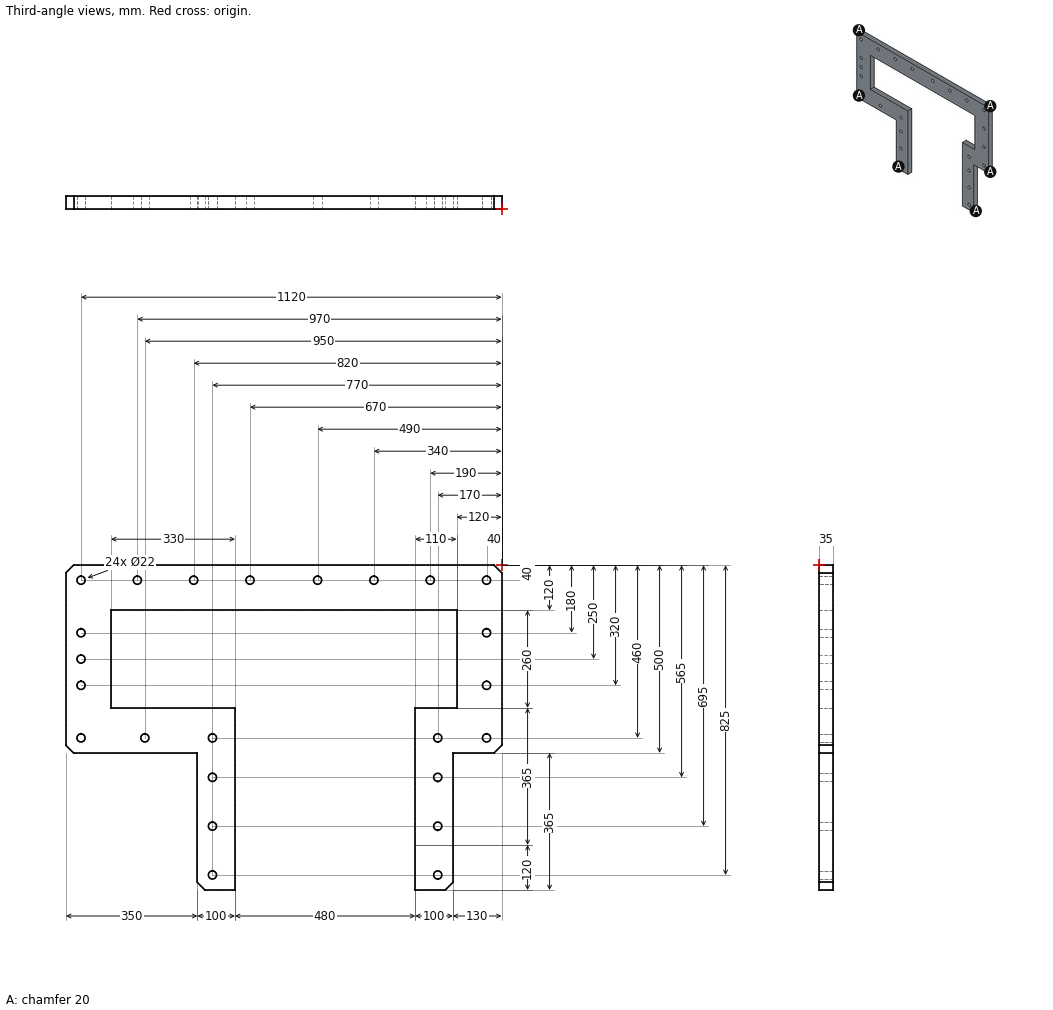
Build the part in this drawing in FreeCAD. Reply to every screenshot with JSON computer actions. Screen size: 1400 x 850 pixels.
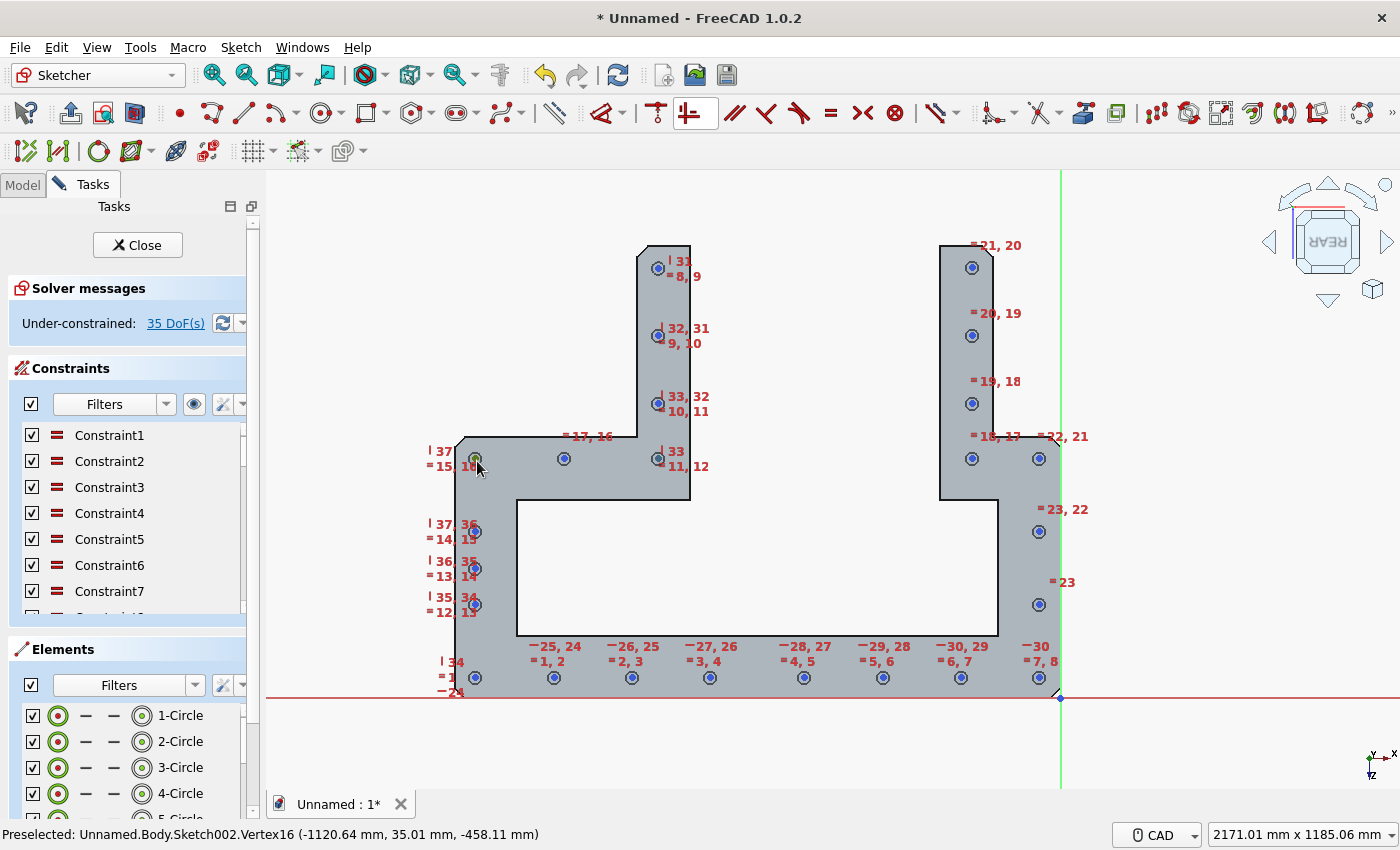
{"action": "key", "text": "h"}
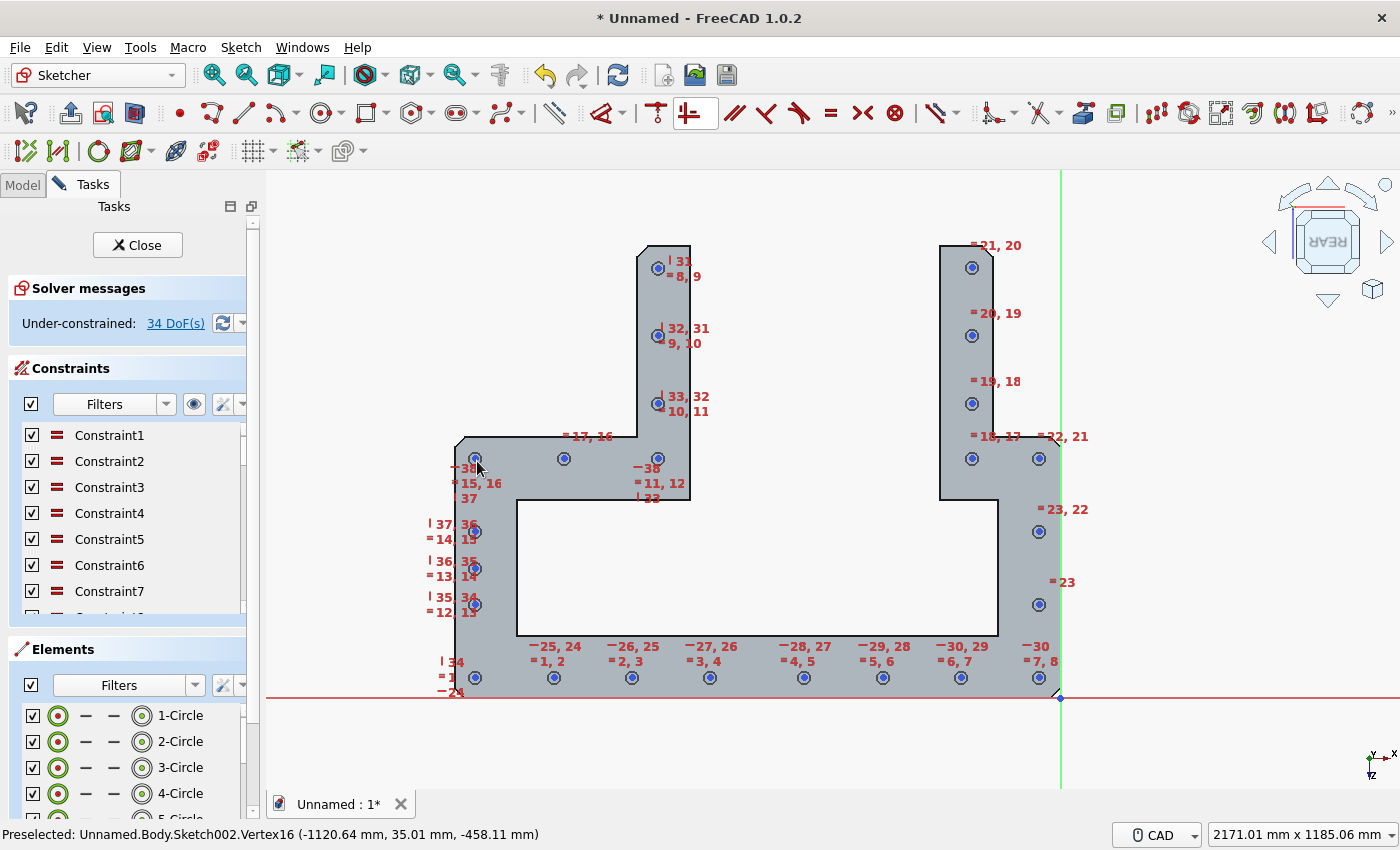
{"action": "left_click", "coordinate": [475, 459]}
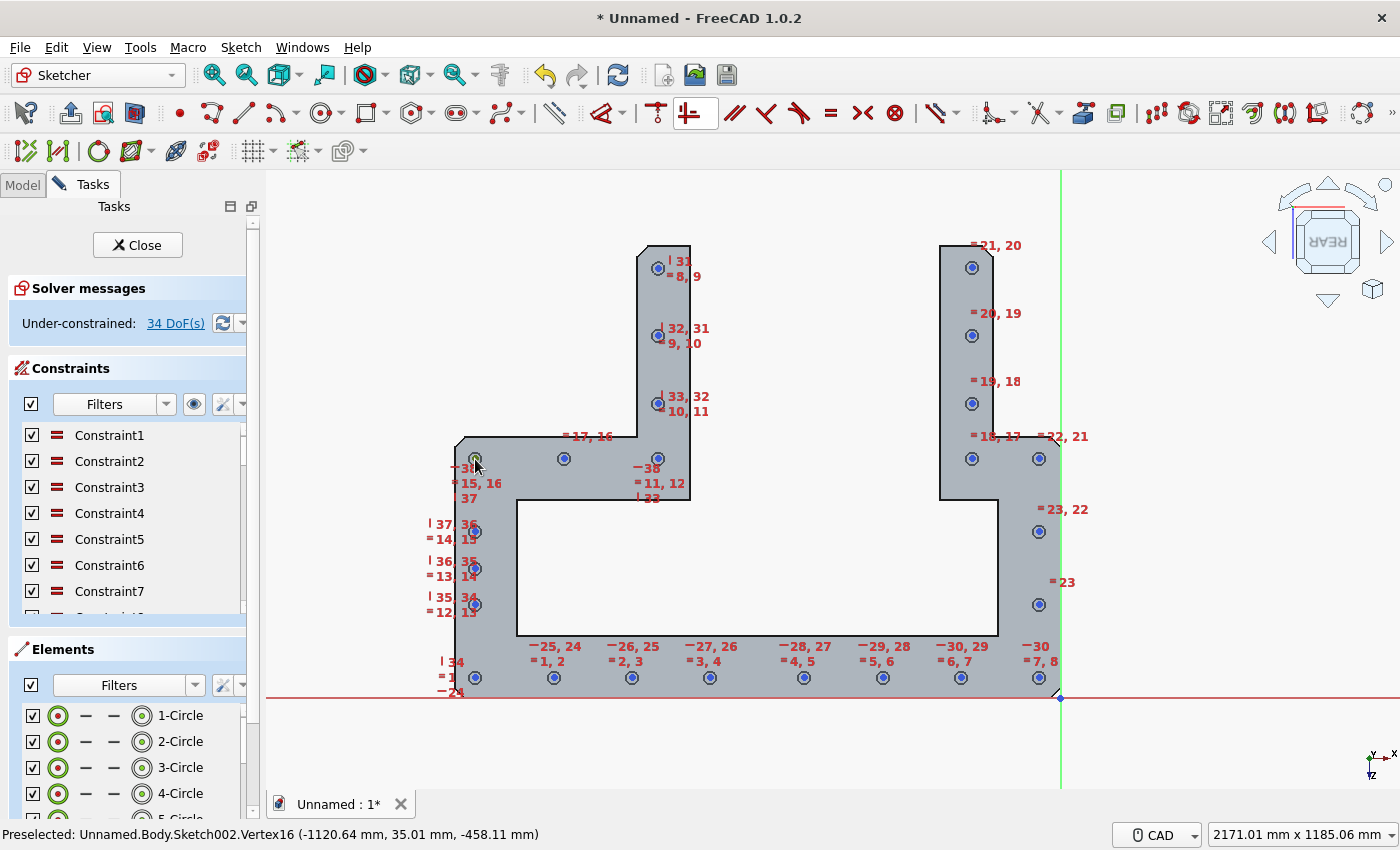
{"action": "left_click", "coordinate": [564, 459]}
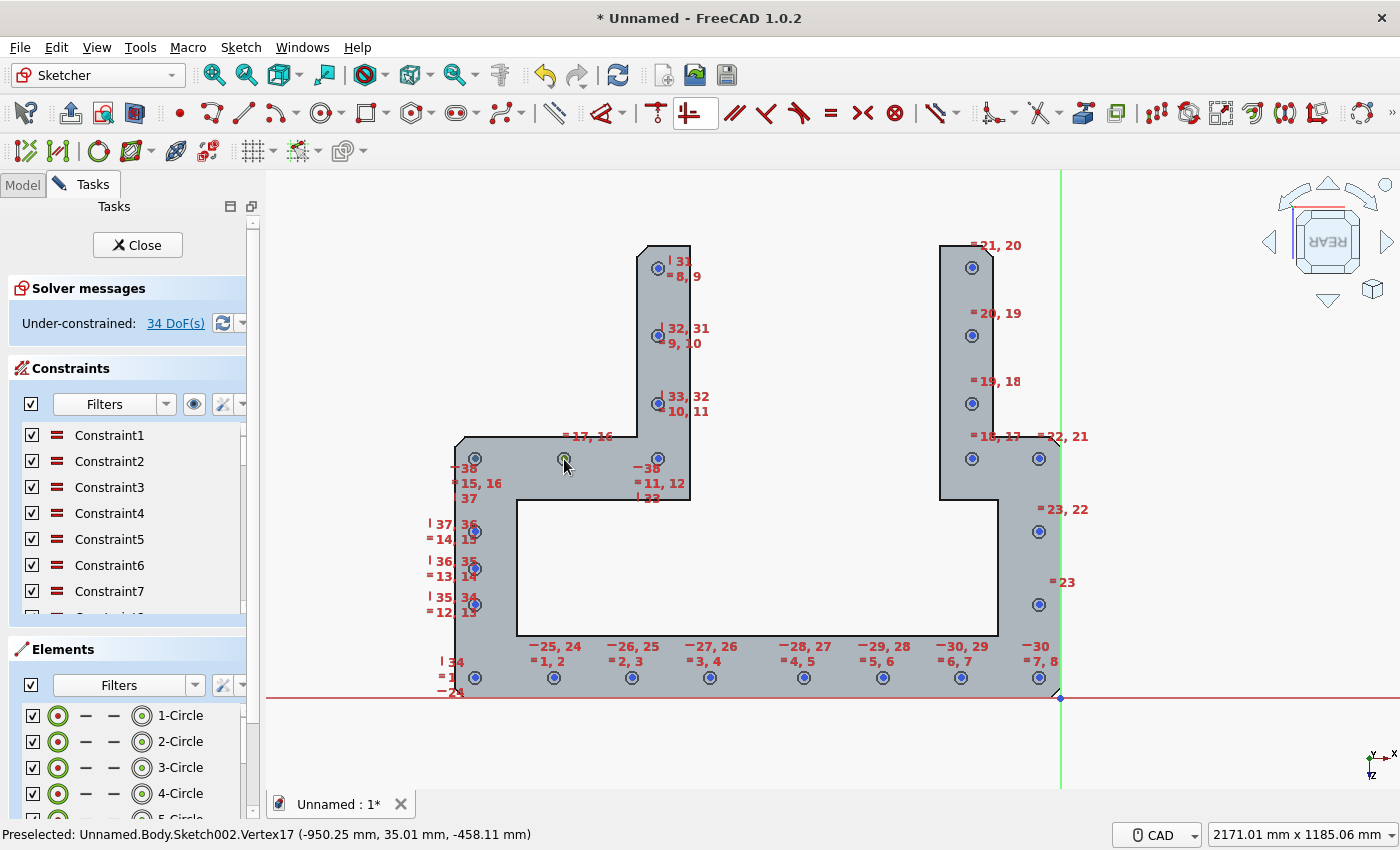
{"action": "key", "text": "h"}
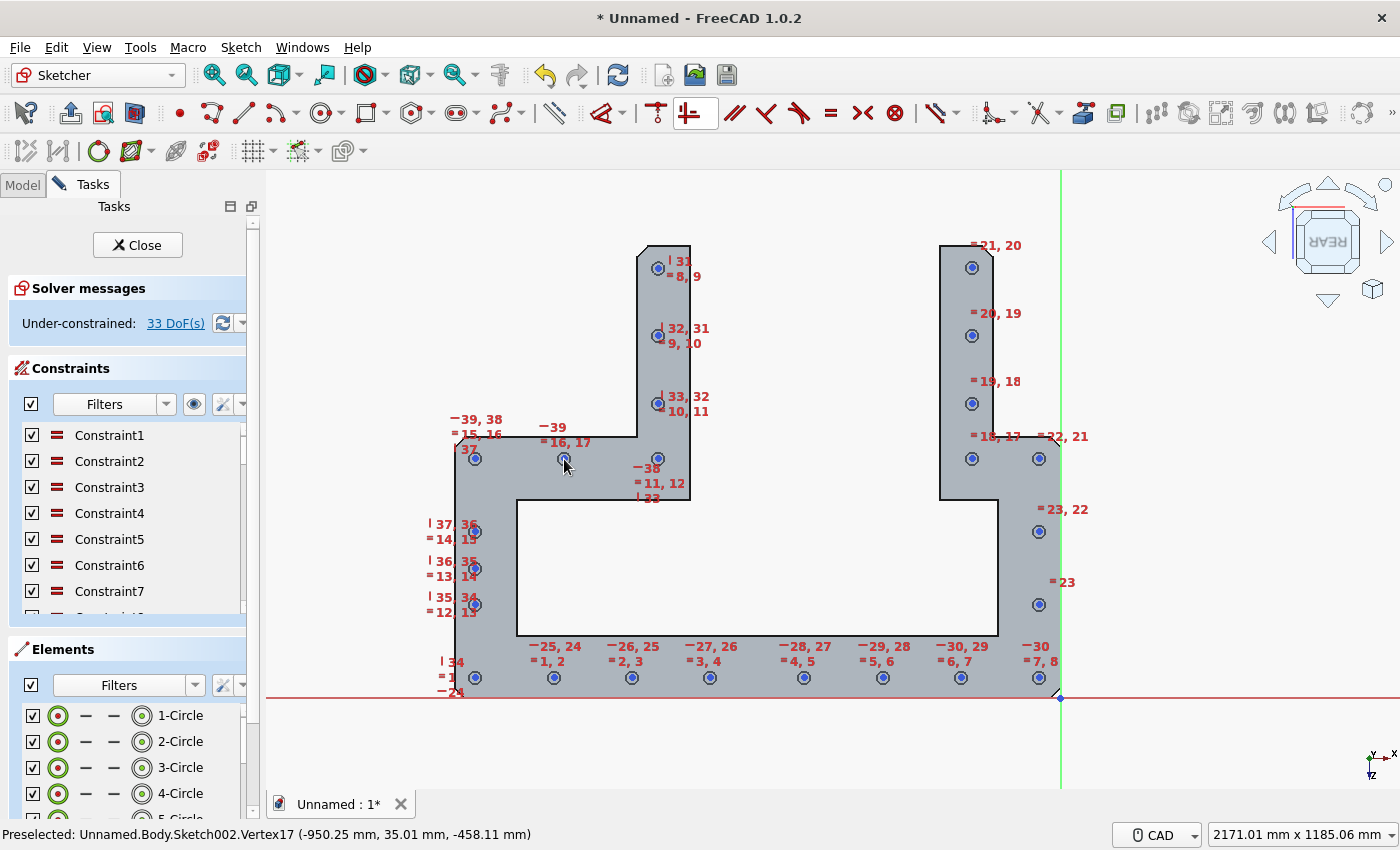
{"action": "left_click", "coordinate": [658, 459]}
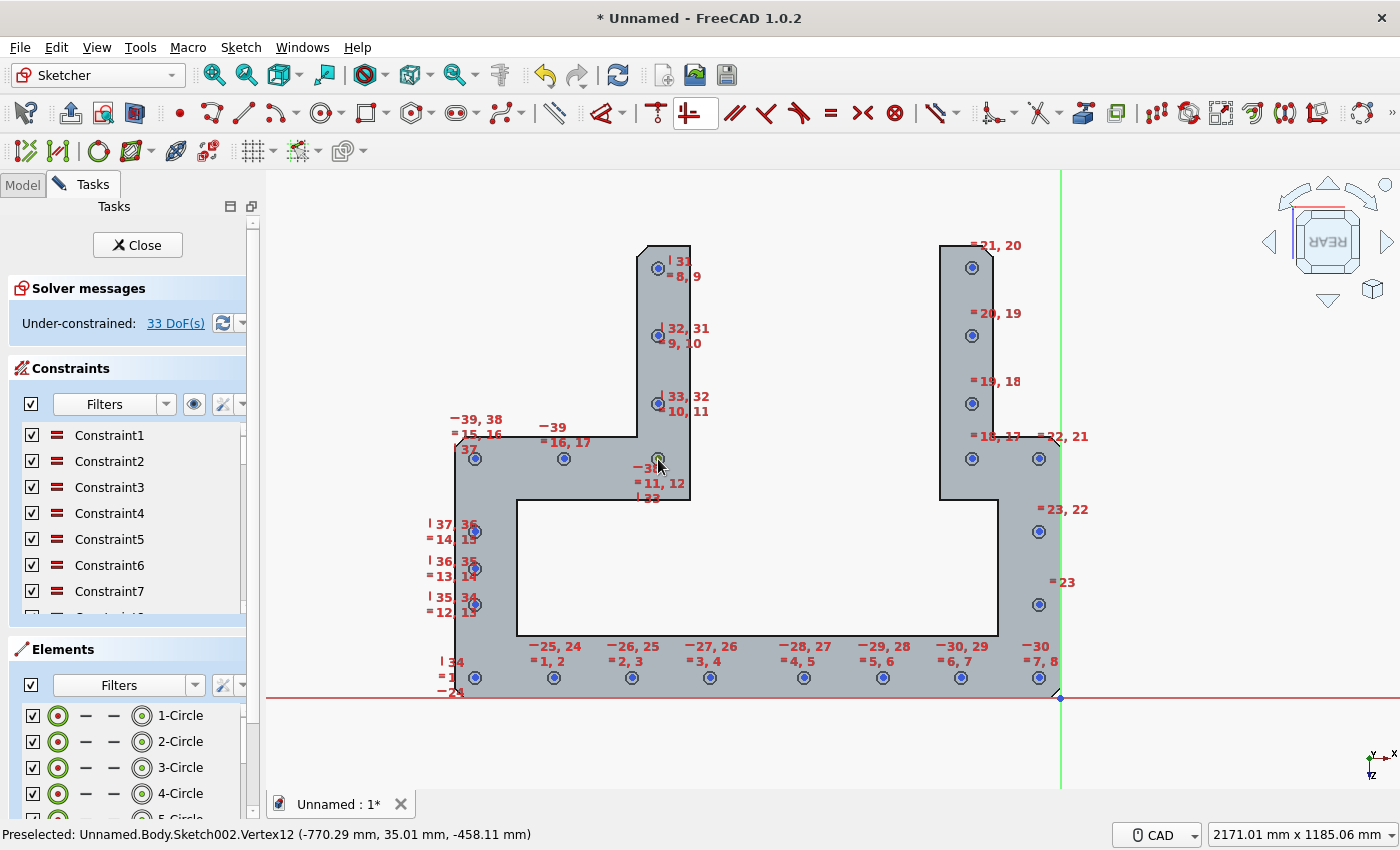
{"action": "left_click", "coordinate": [972, 459]}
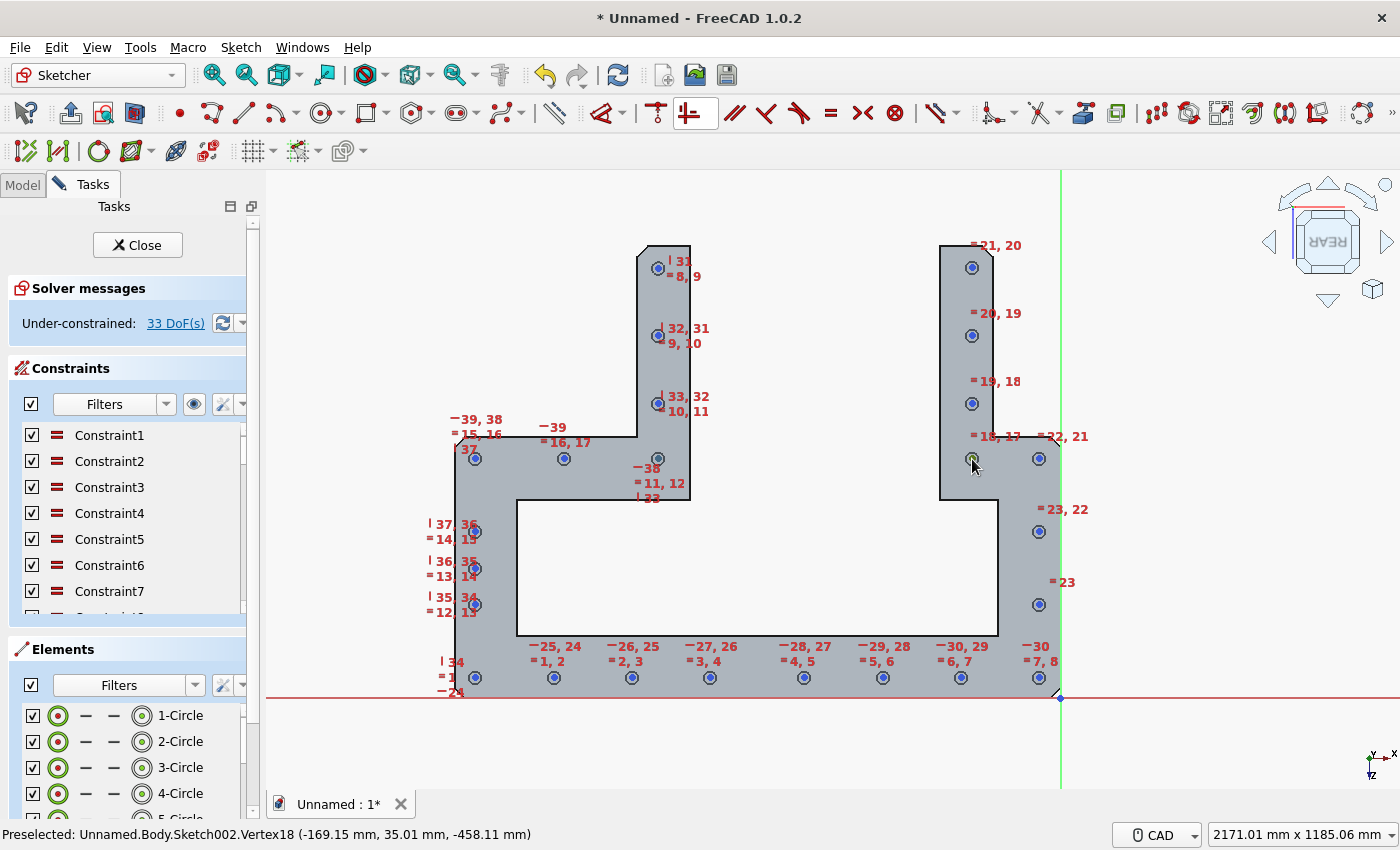
{"action": "left_click", "coordinate": [712, 114]}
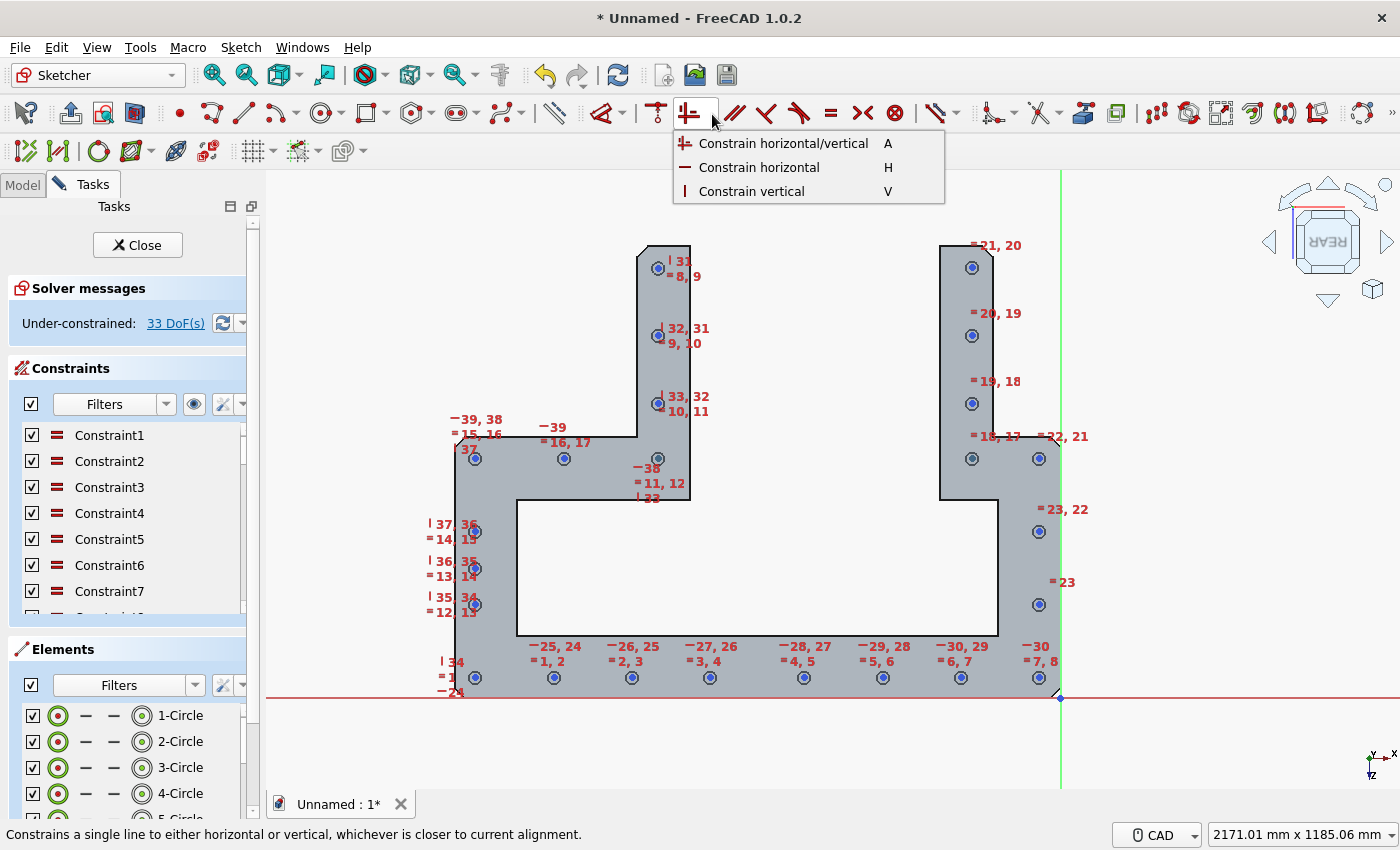
{"action": "left_click", "coordinate": [809, 167]}